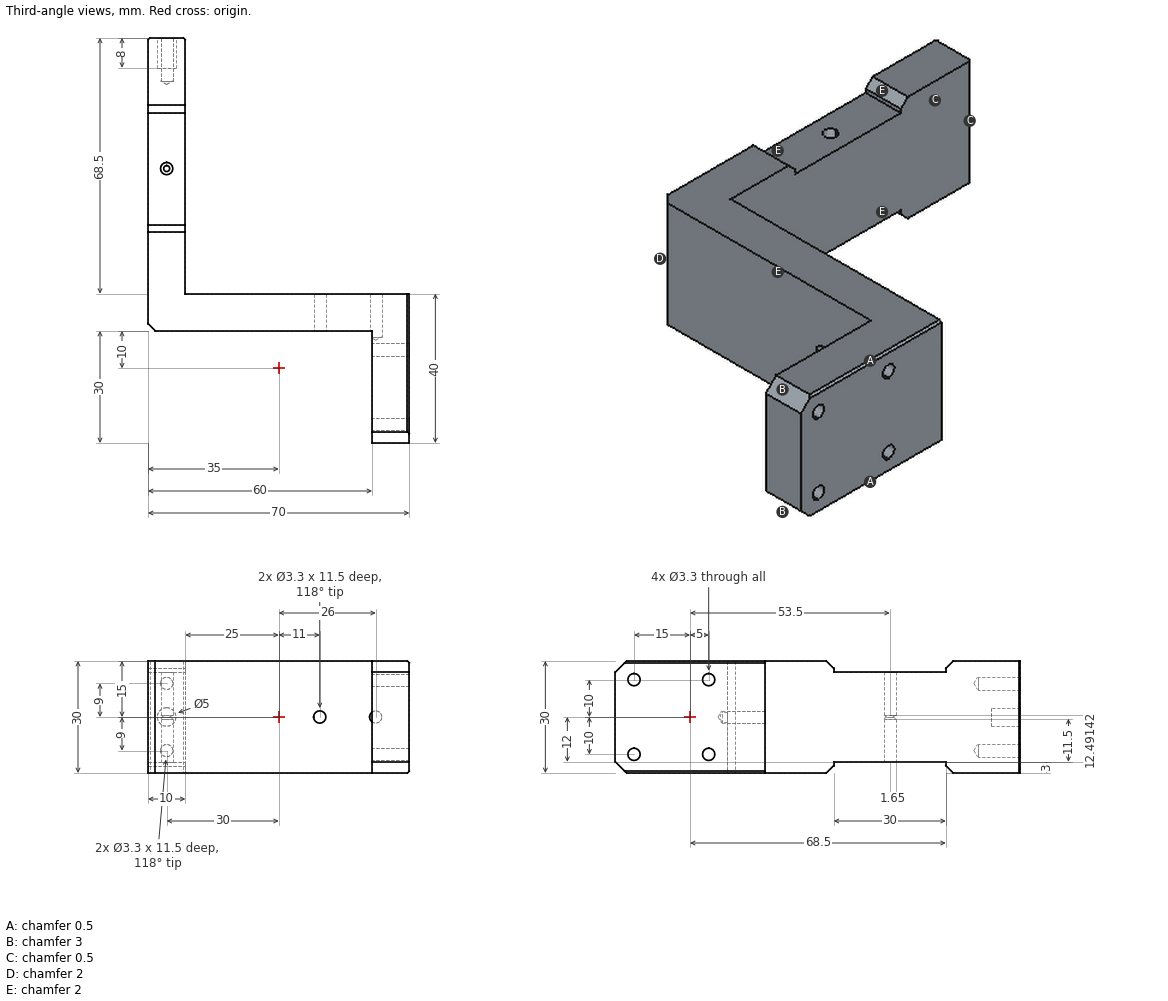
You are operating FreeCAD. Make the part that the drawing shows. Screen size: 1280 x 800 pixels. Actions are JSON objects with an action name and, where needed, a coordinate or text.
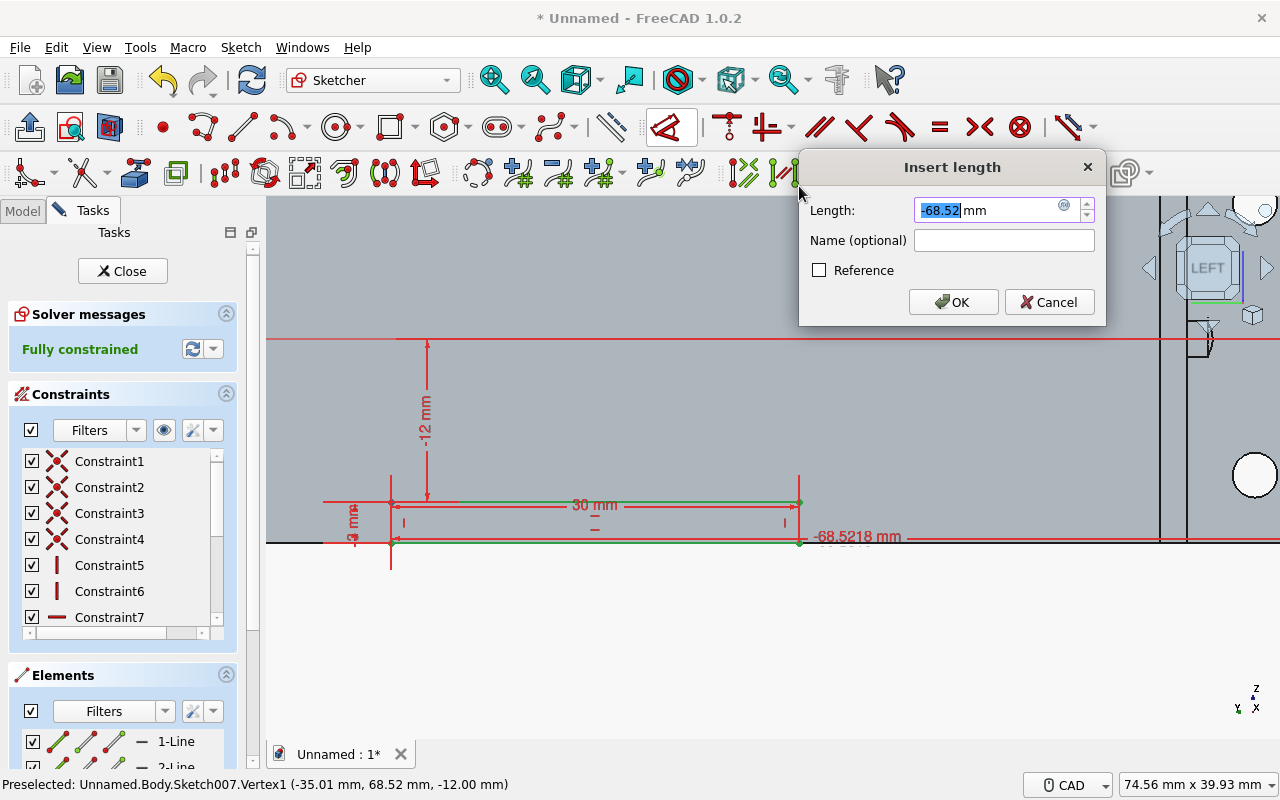
{"action": "type", "text": "-68.5"}
{"action": "key", "text": "Return"}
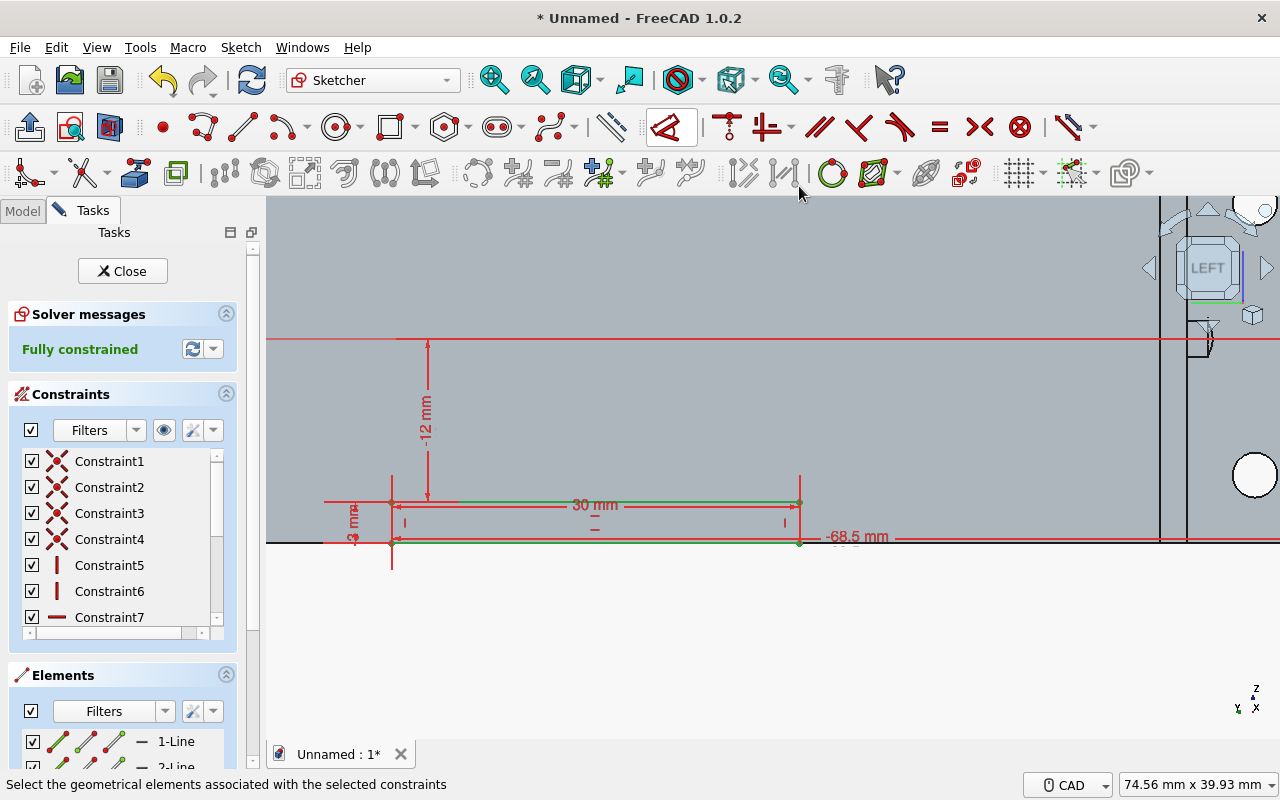
{"action": "left_click", "coordinate": [123, 271]}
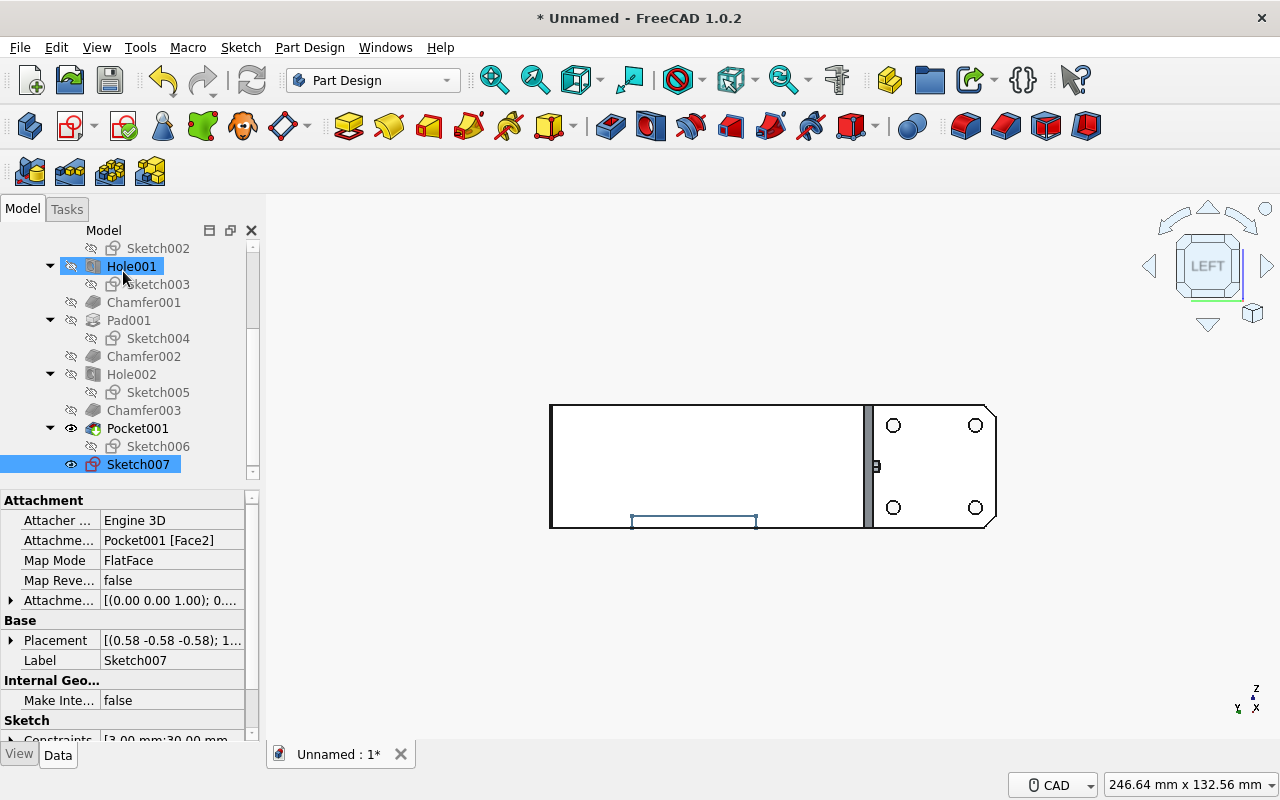
{"action": "left_click", "coordinate": [612, 126]}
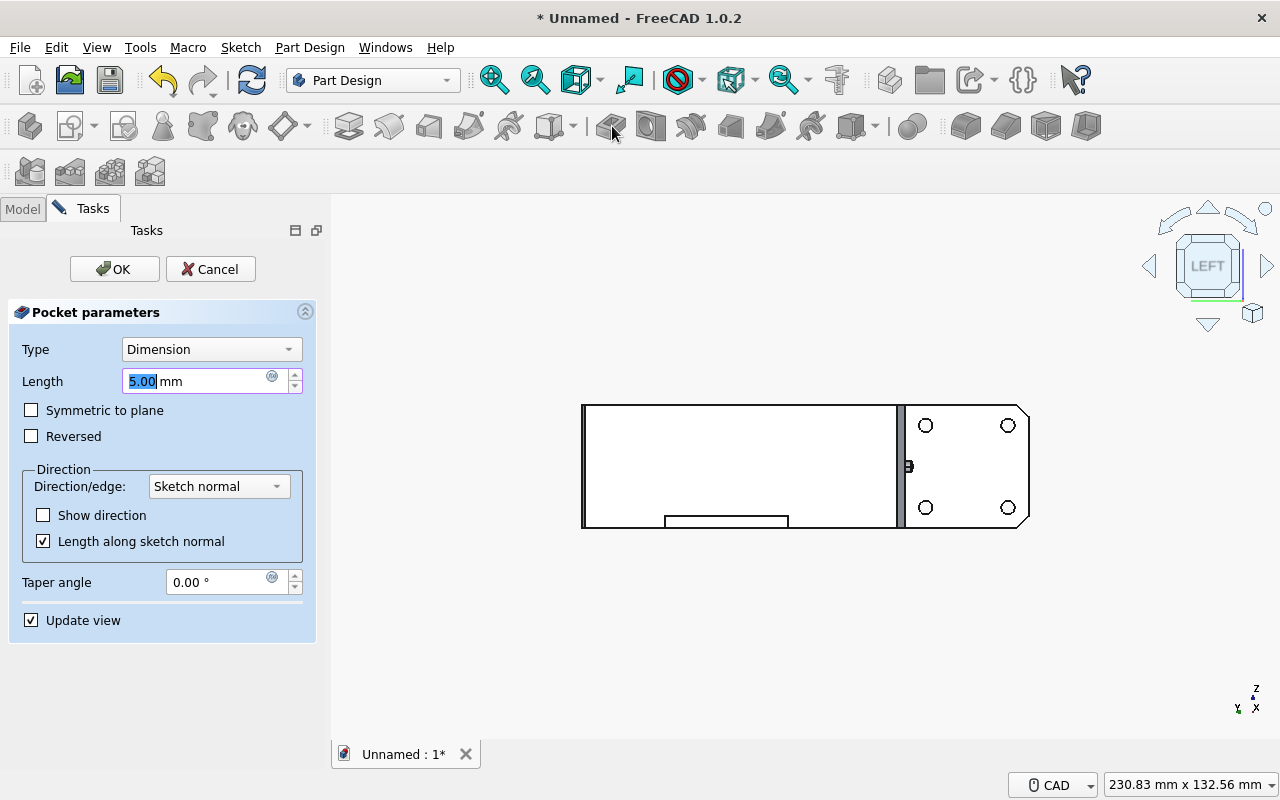
{"action": "left_click", "coordinate": [212, 350]}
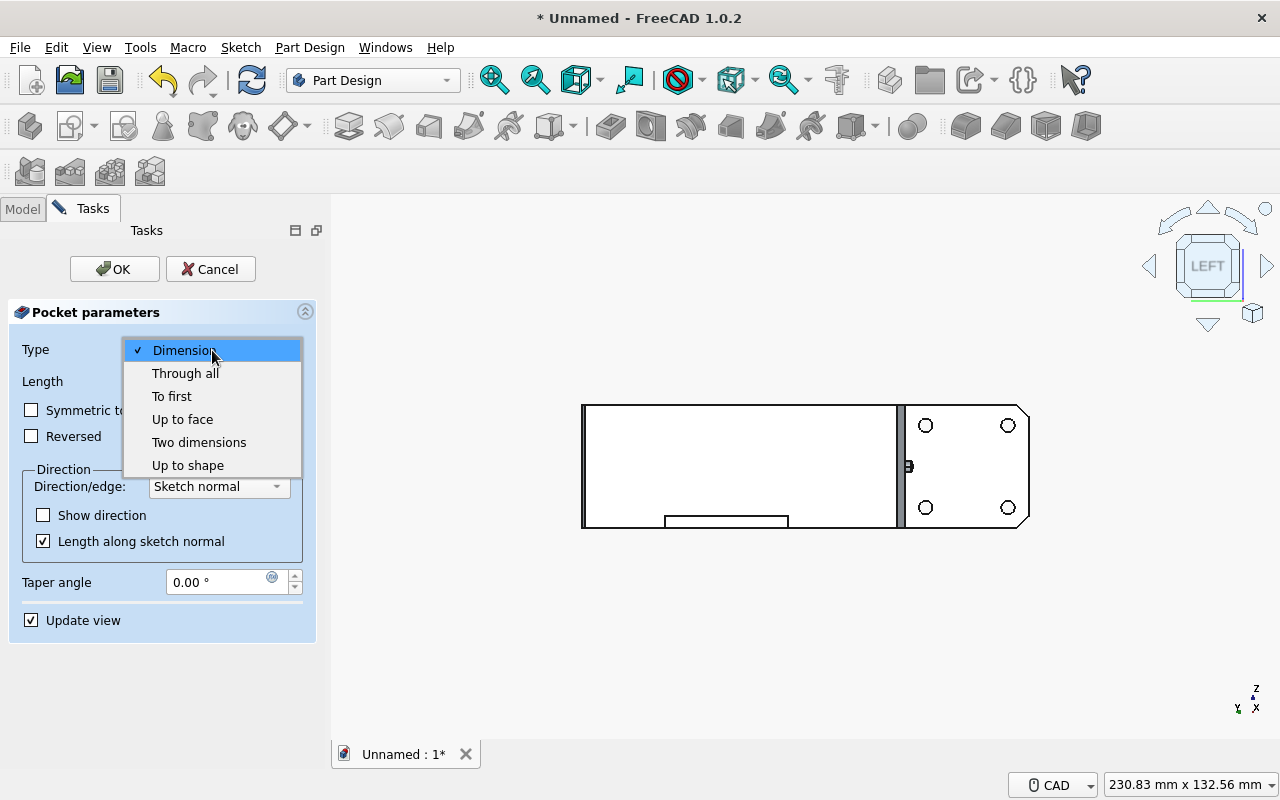
{"action": "left_click", "coordinate": [212, 374]}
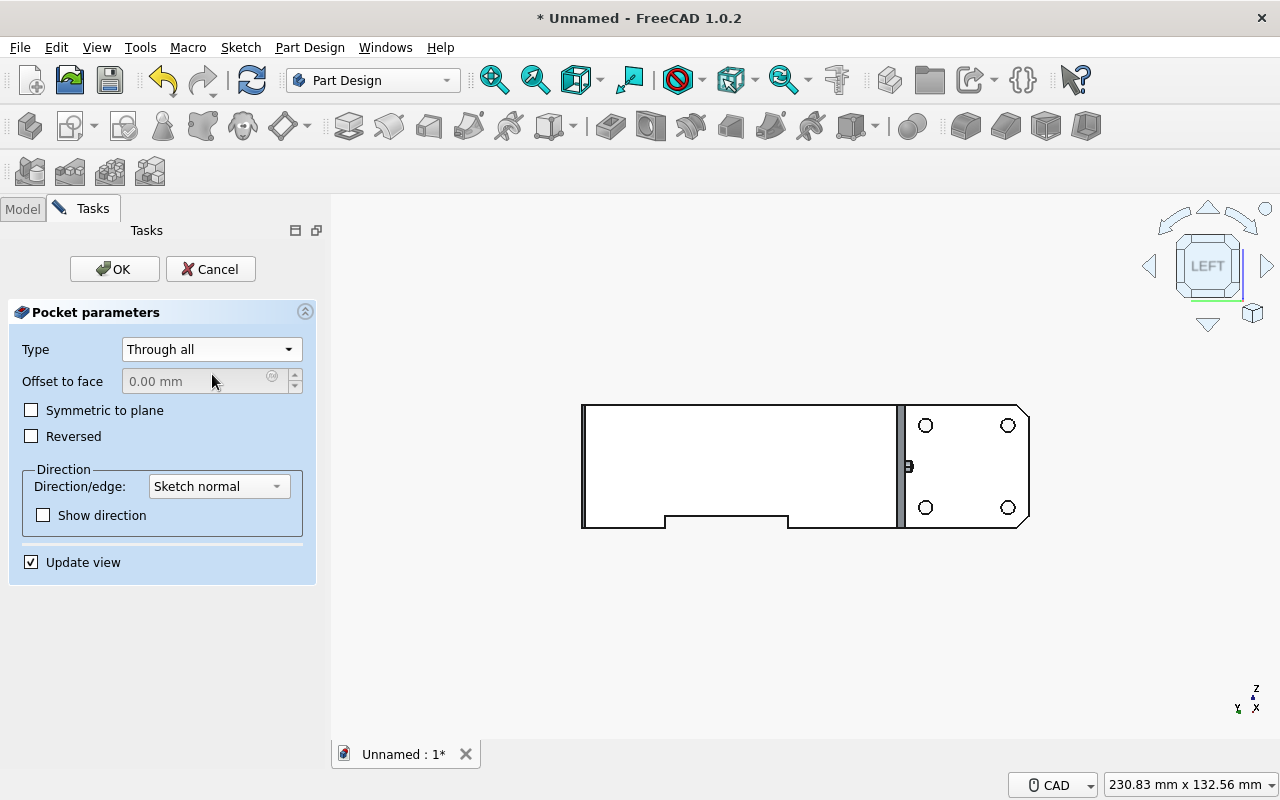
{"action": "left_click", "coordinate": [115, 269]}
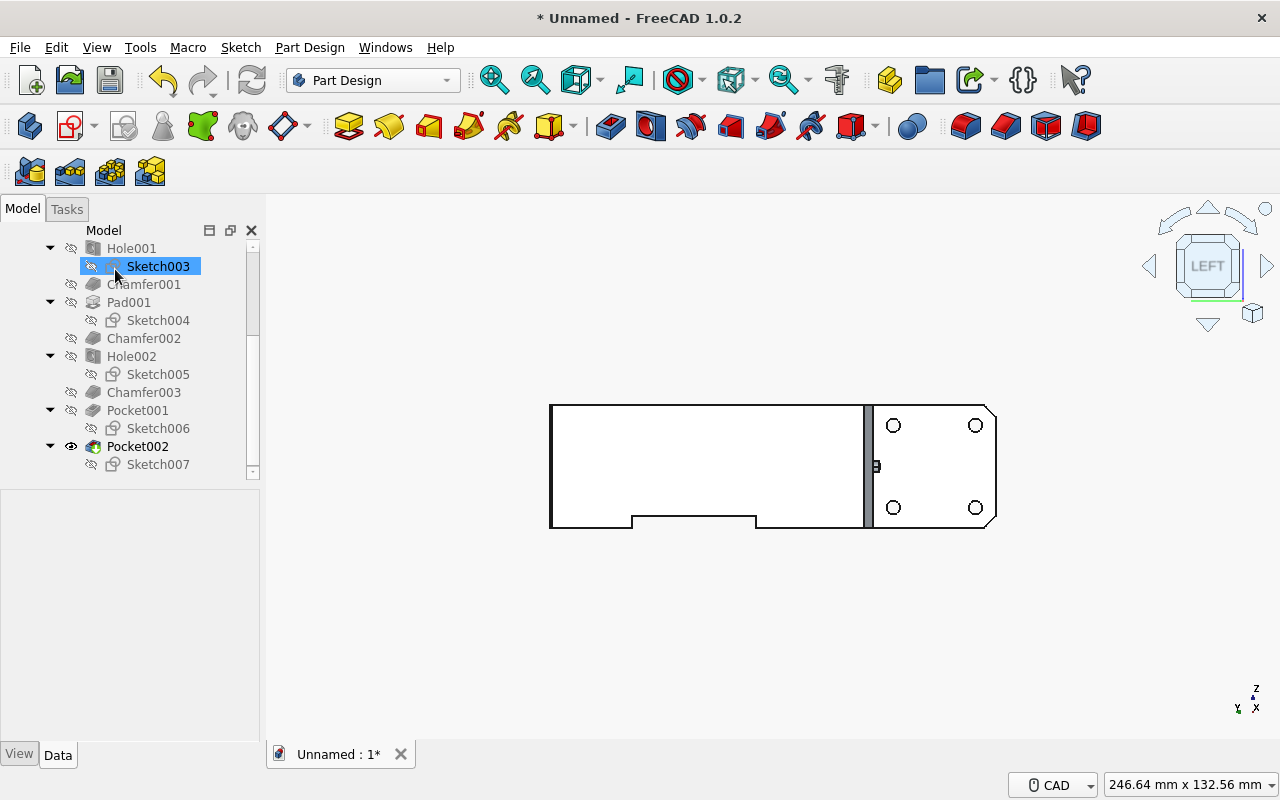
{"action": "left_click", "coordinate": [496, 80]}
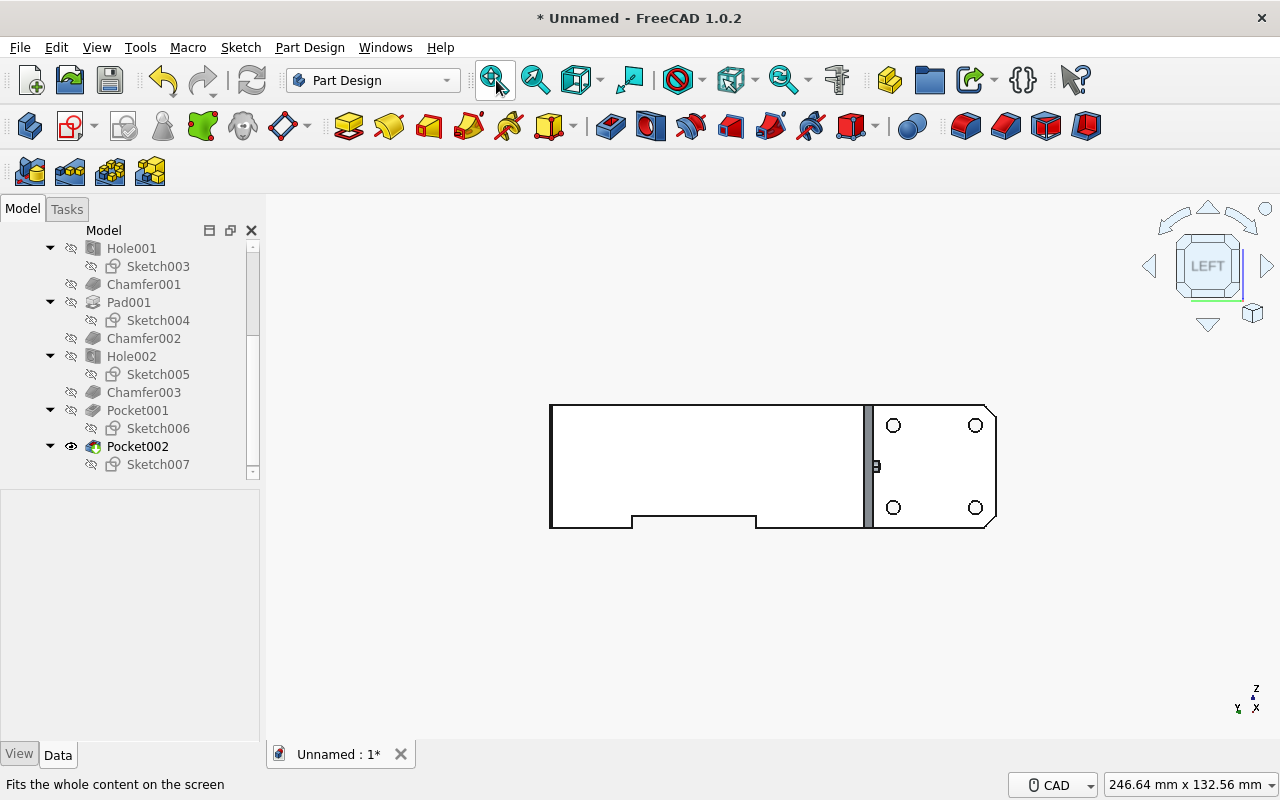
{"action": "scroll", "coordinate": [140, 352], "scroll_direction": "down", "scroll_amount": 3}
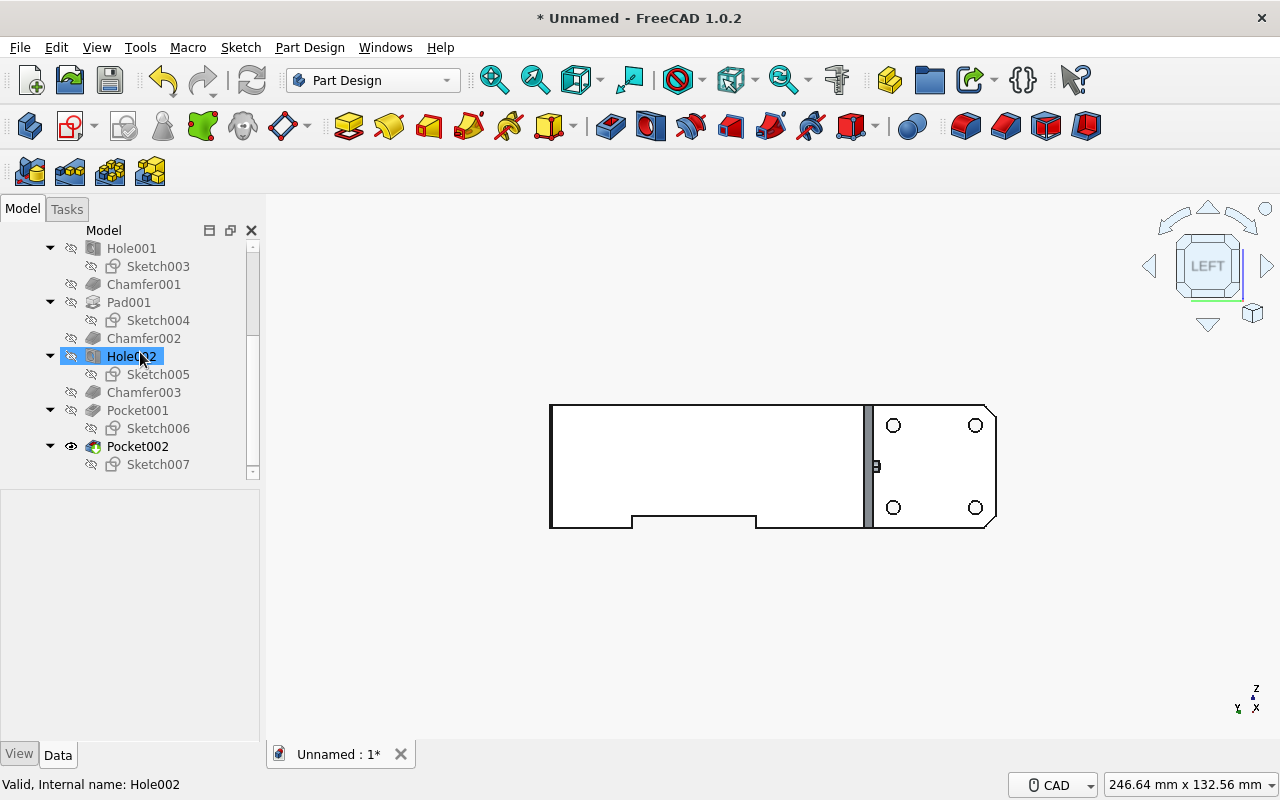
{"action": "scroll", "coordinate": [140, 352], "scroll_direction": "up", "scroll_amount": 15}